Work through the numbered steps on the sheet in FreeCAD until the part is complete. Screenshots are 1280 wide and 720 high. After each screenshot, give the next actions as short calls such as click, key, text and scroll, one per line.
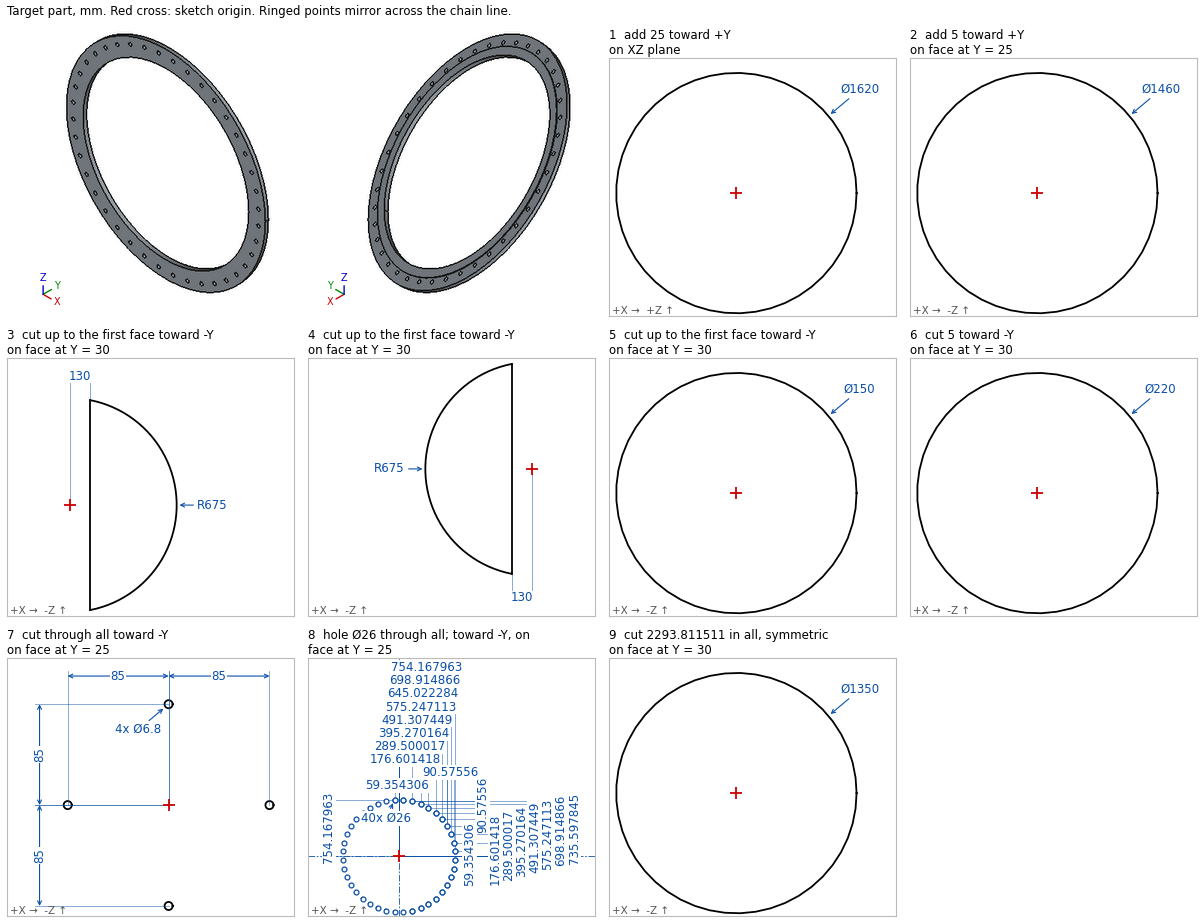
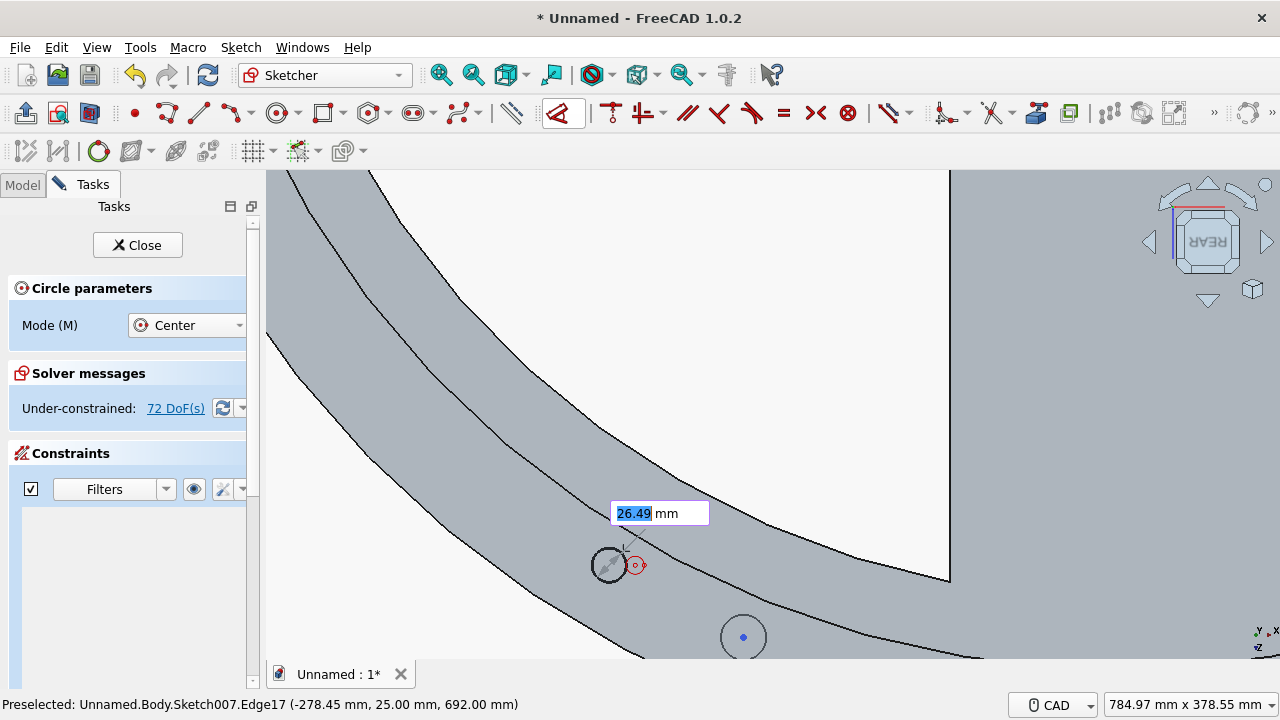
click(619, 548)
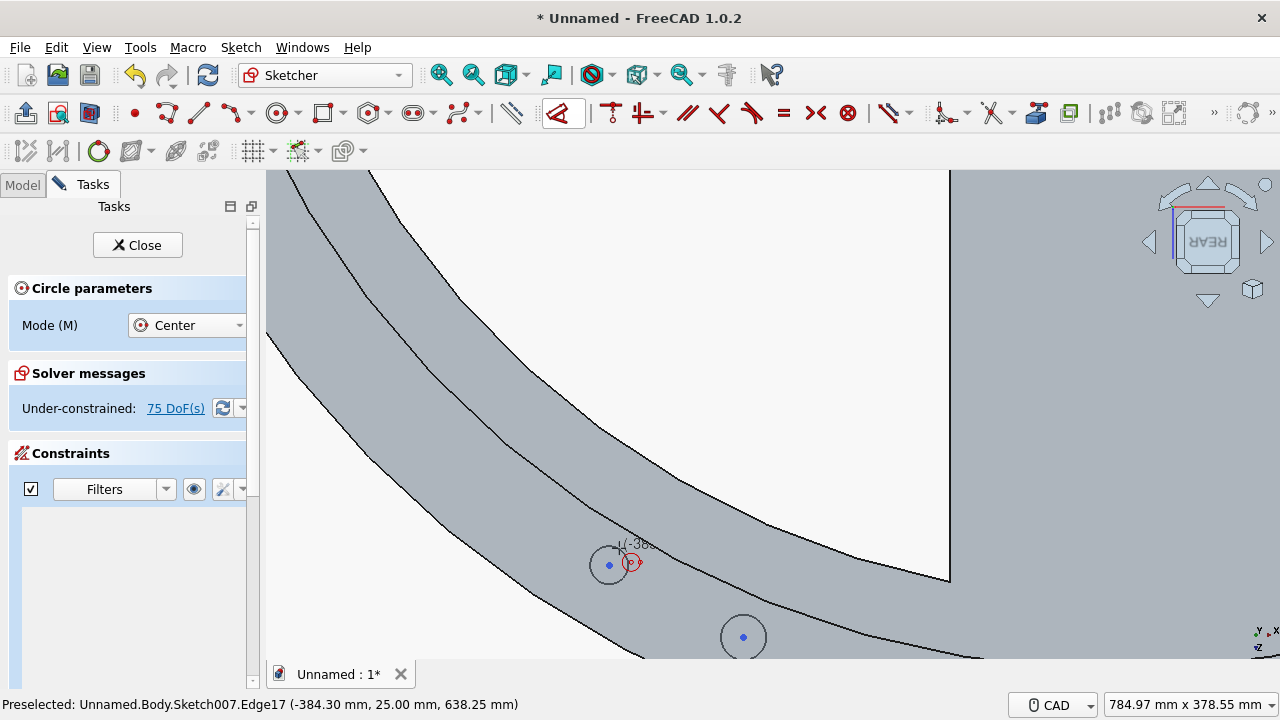
scroll(483, 469, up, 2)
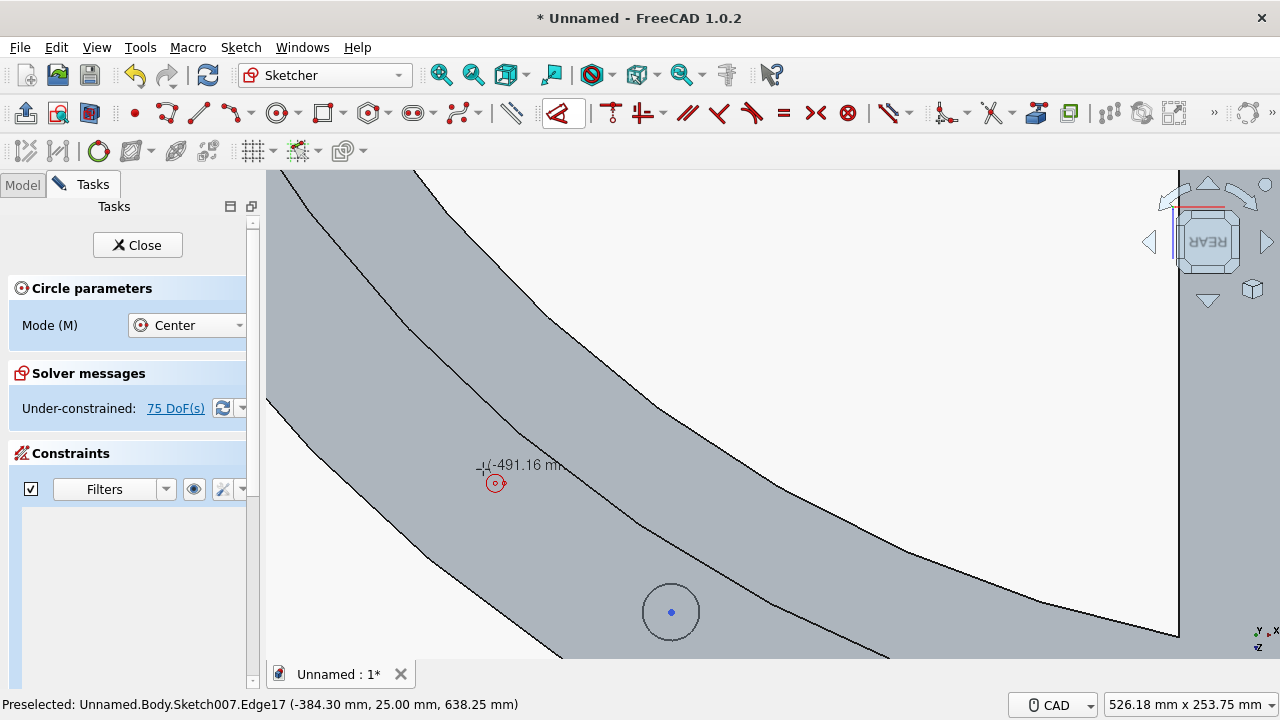
scroll(614, 546, down, 11)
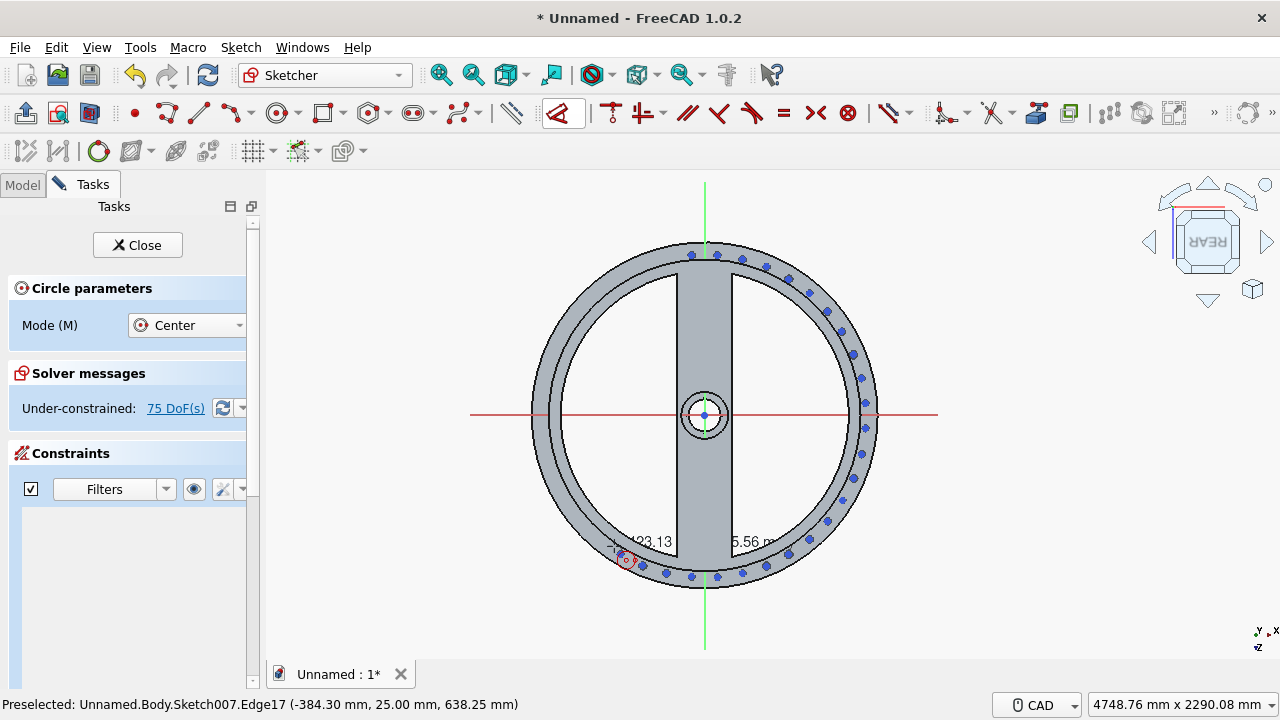
click(600, 538)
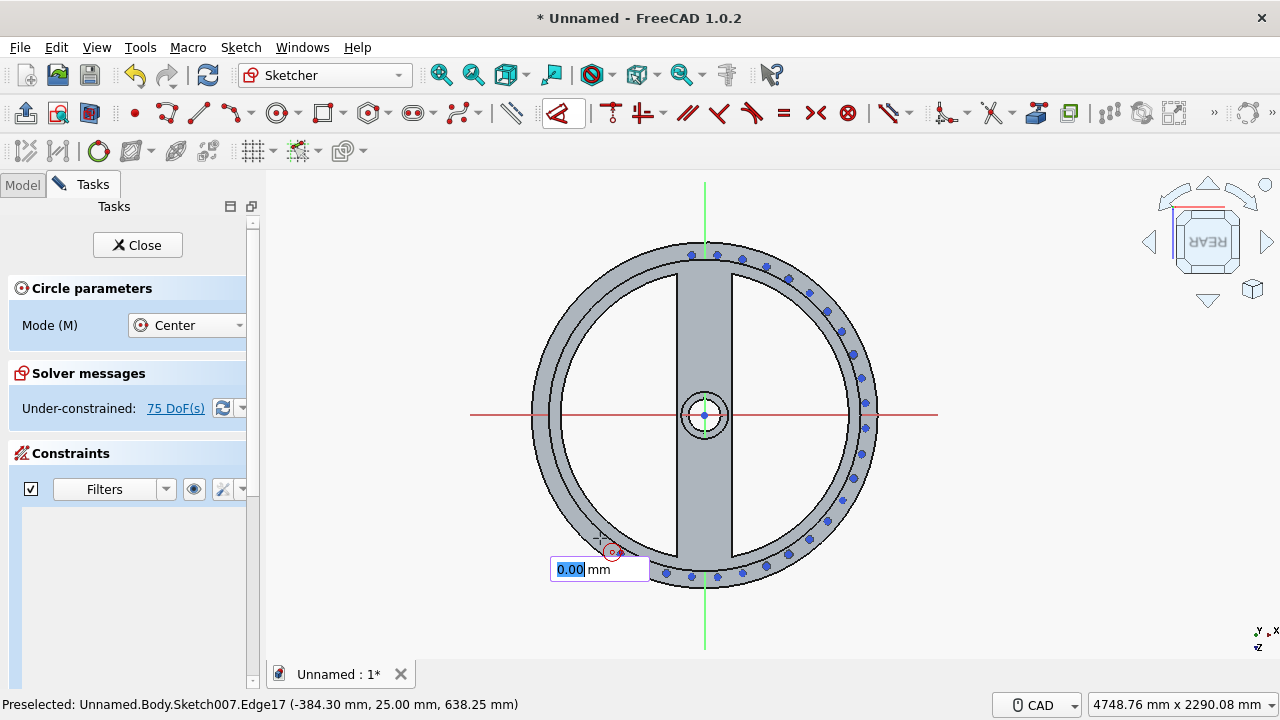
scroll(602, 536, up, 9)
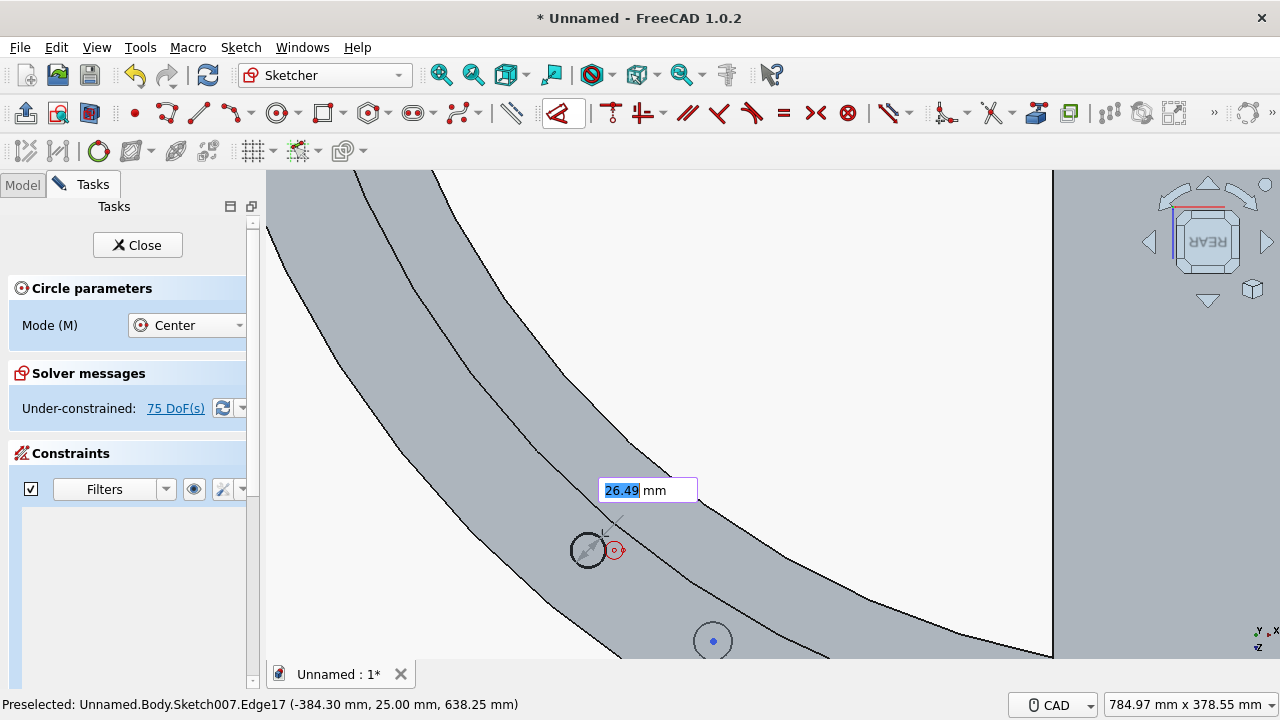
click(599, 534)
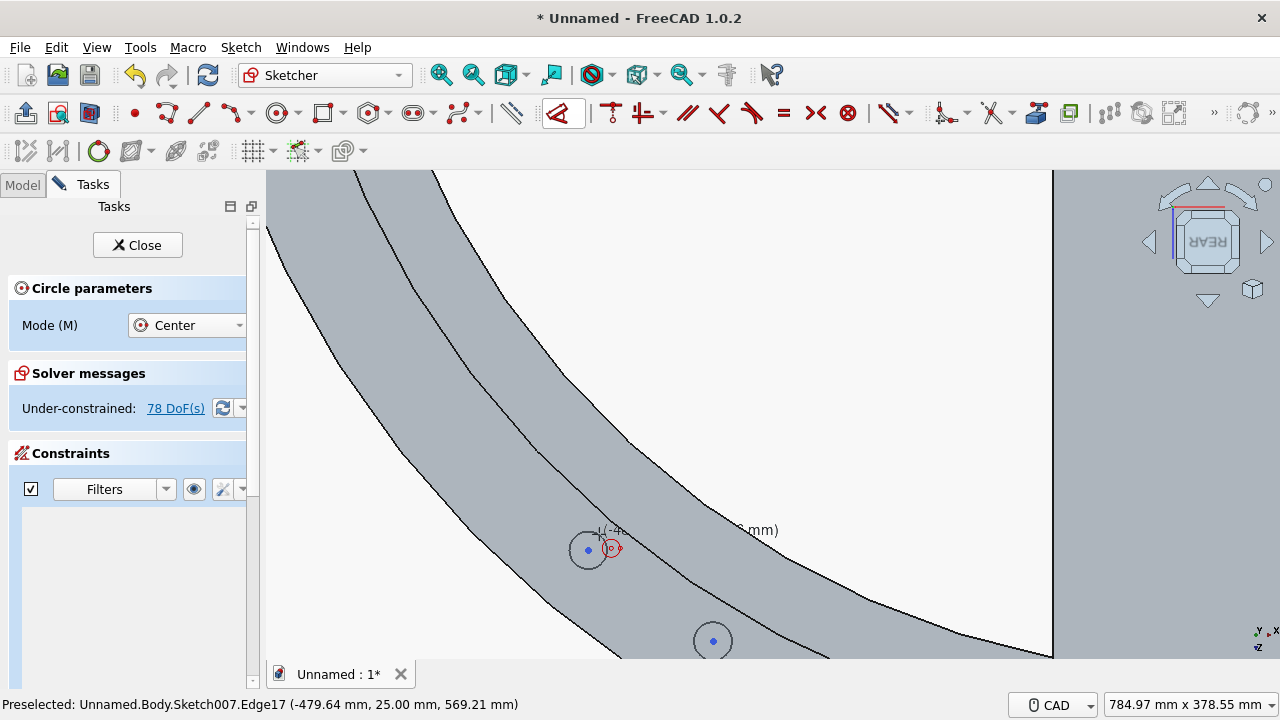
scroll(478, 437, up, 2)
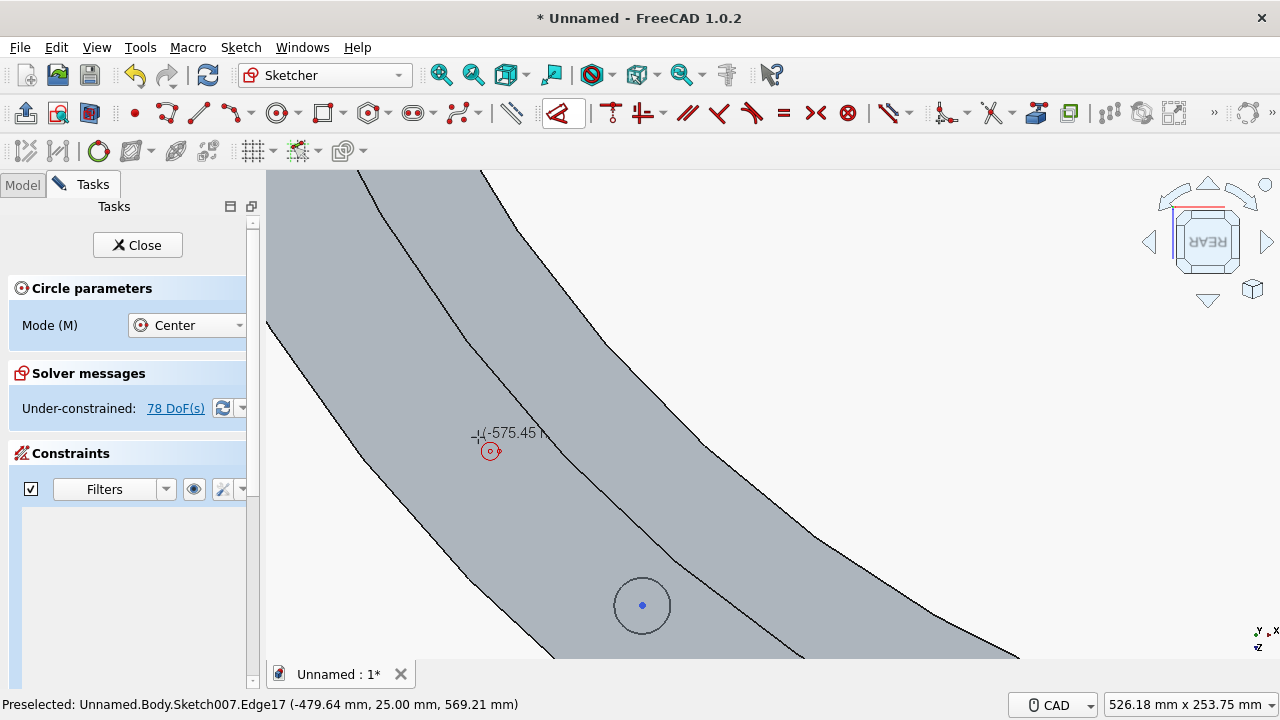
scroll(595, 530, down, 11)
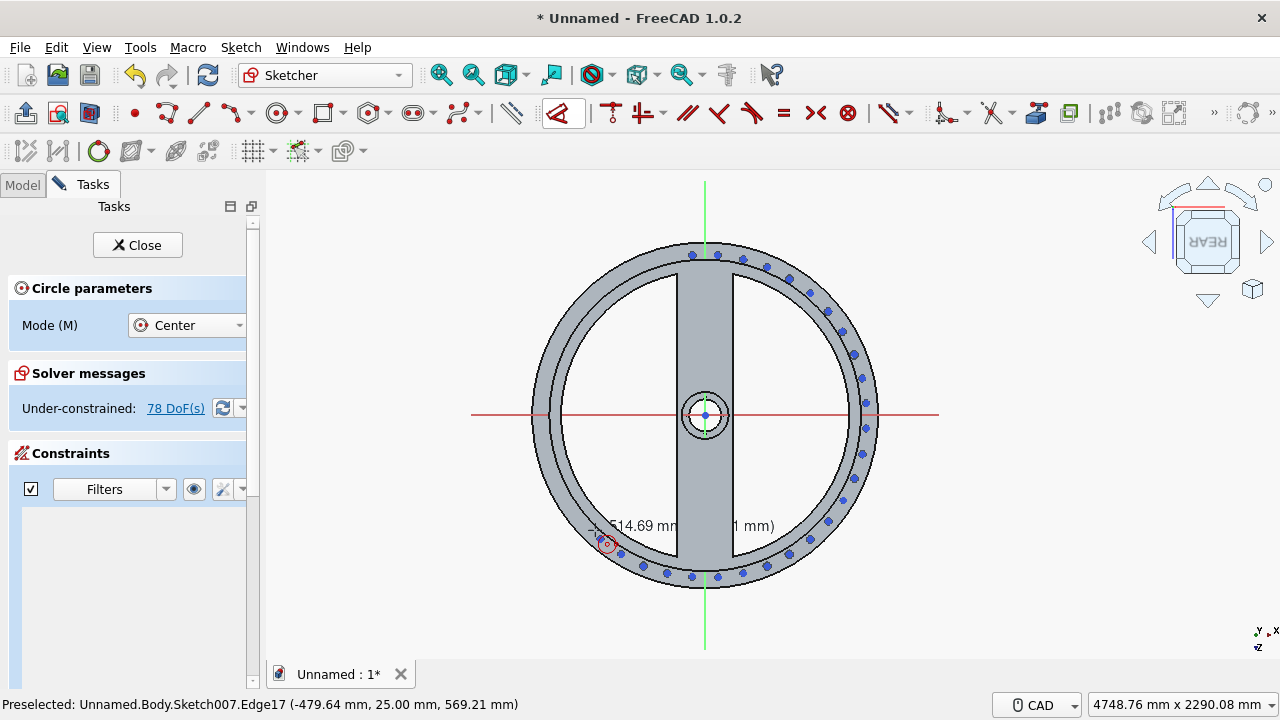
click(582, 520)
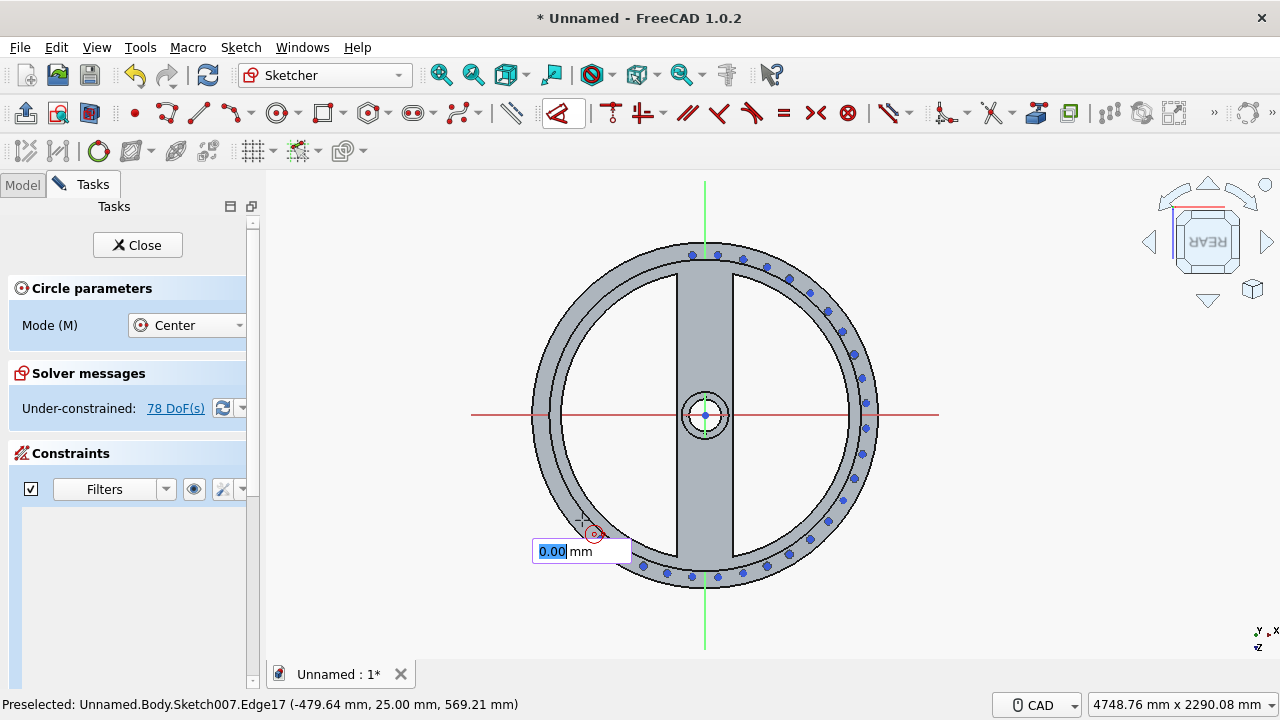
scroll(584, 518, up, 9)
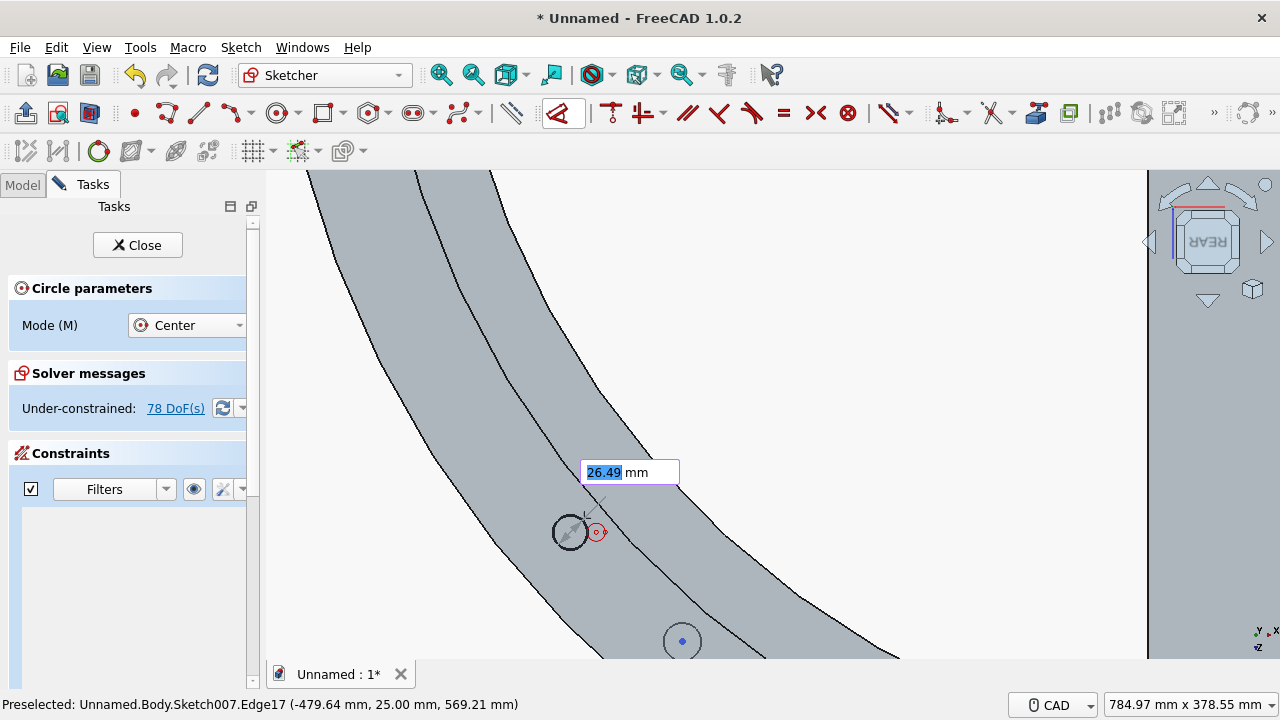
click(584, 517)